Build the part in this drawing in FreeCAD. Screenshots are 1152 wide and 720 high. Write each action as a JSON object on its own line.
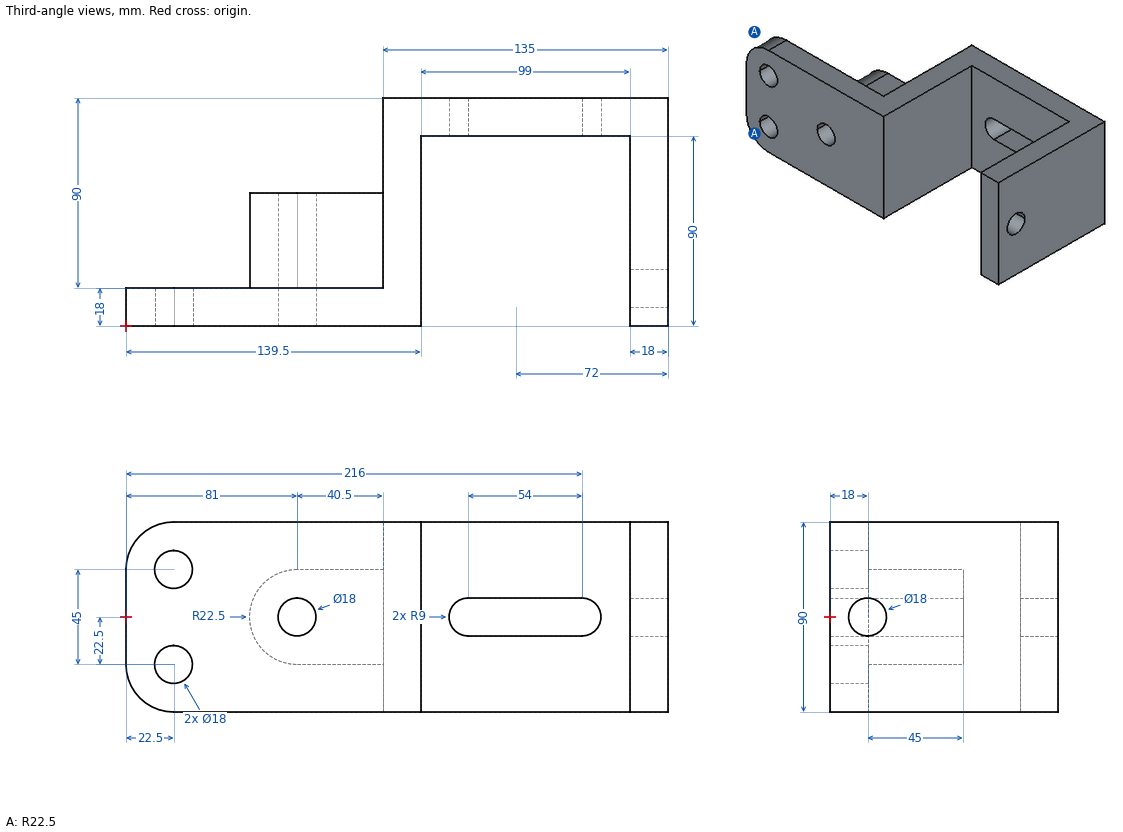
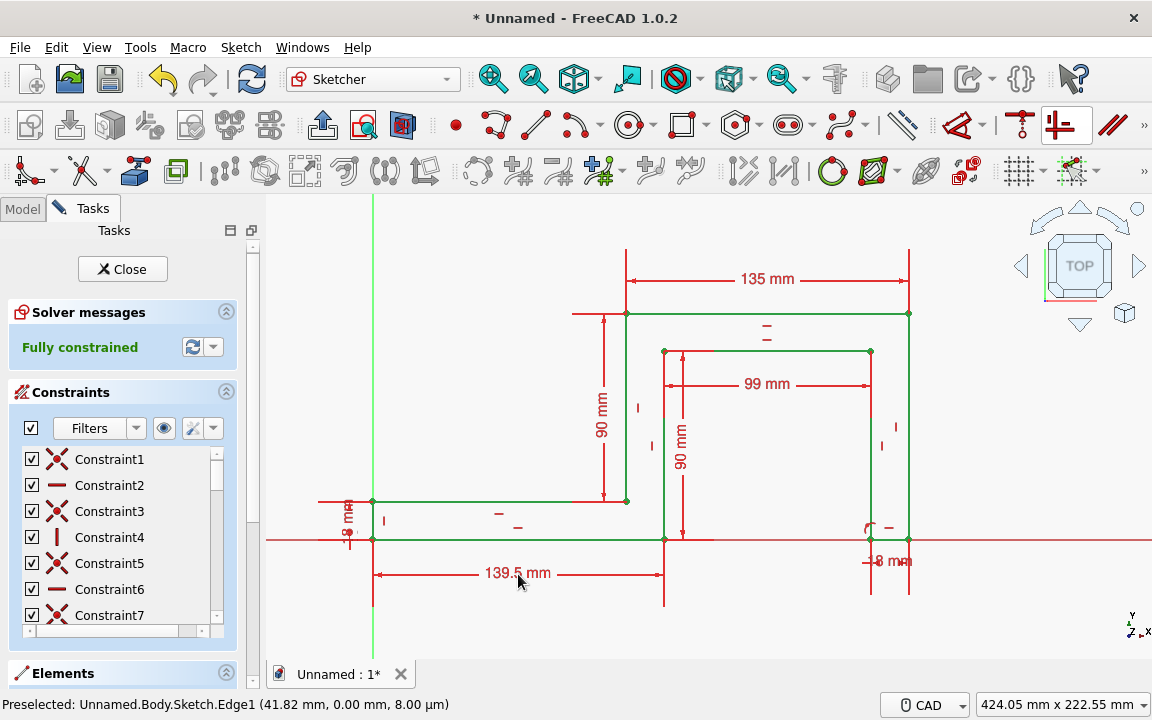
{"action": "left_click", "coordinate": [123, 269]}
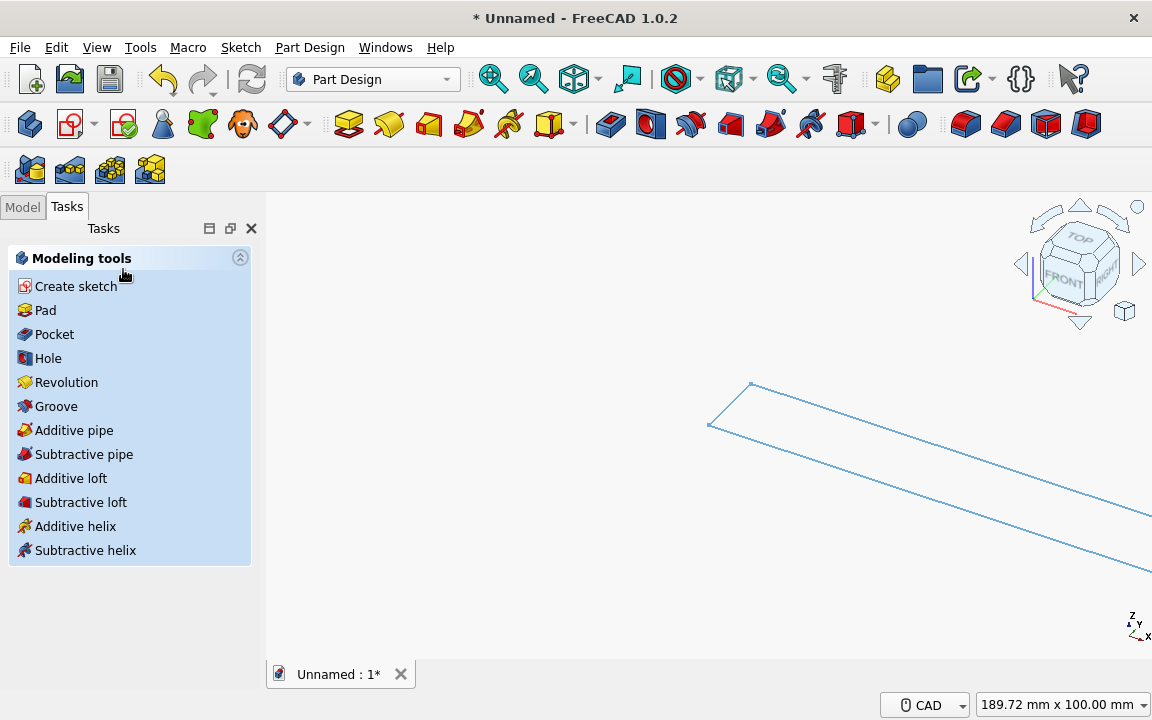
{"action": "left_click", "coordinate": [350, 124]}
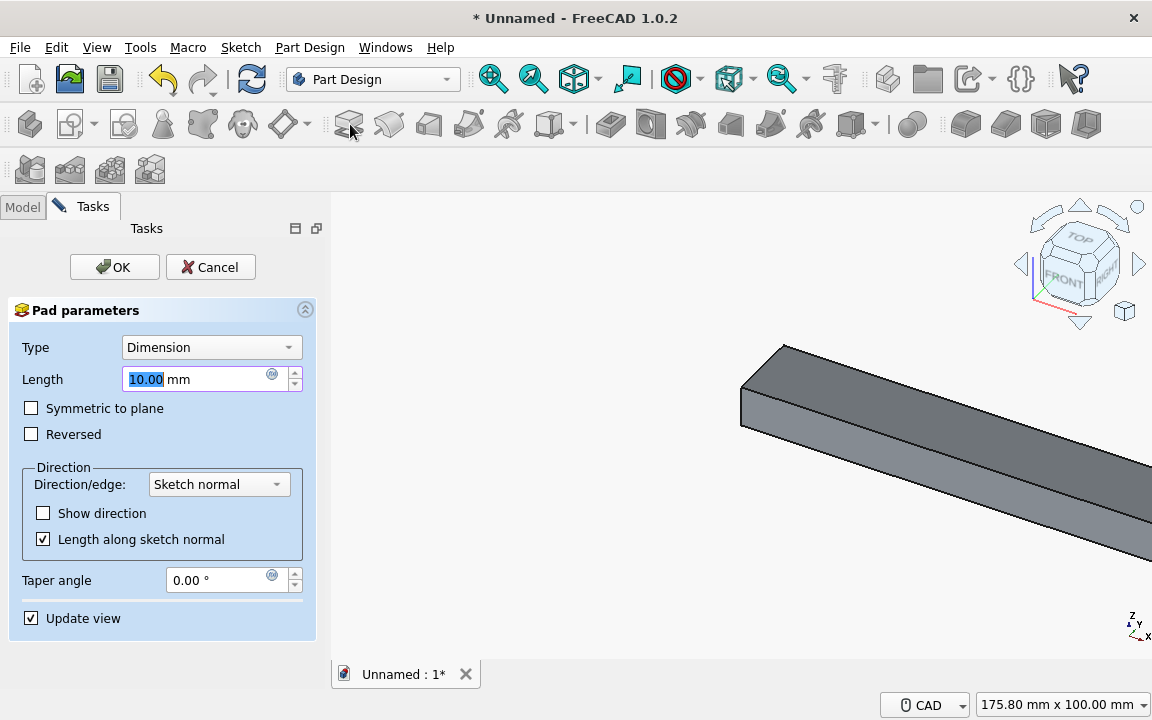
{"action": "type", "text": "90"}
{"action": "key", "text": "Tab"}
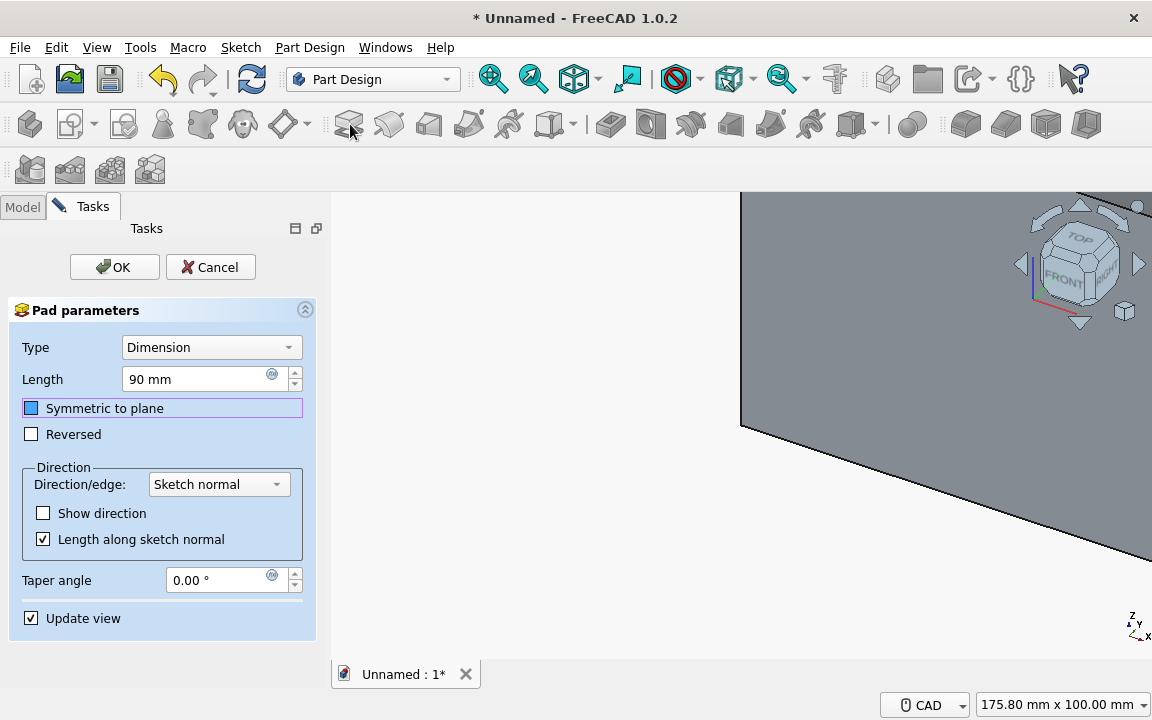
{"action": "left_click", "coordinate": [30, 408]}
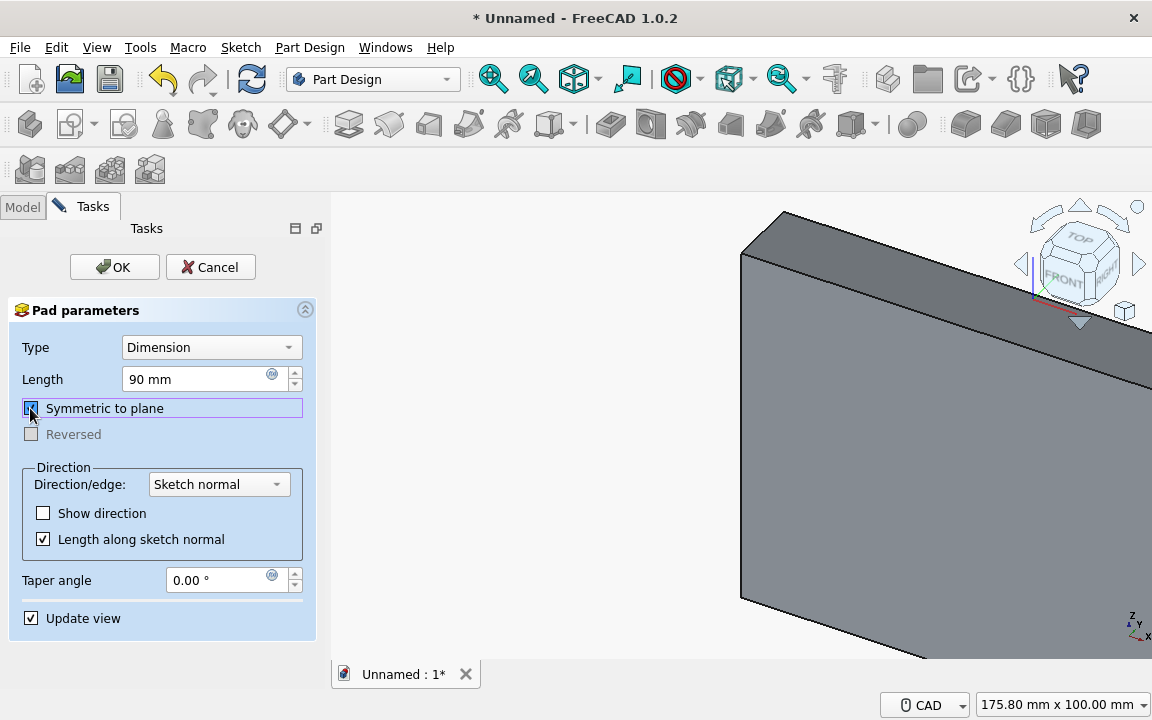
{"action": "left_click", "coordinate": [115, 267]}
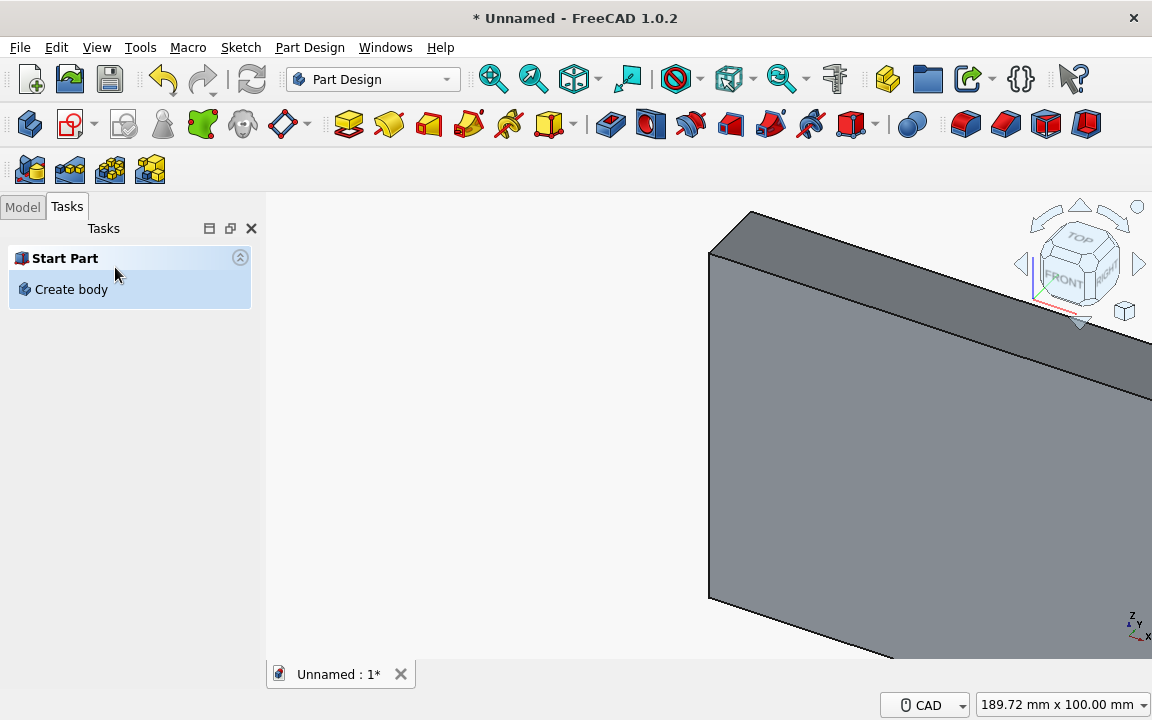
{"action": "left_click", "coordinate": [494, 80]}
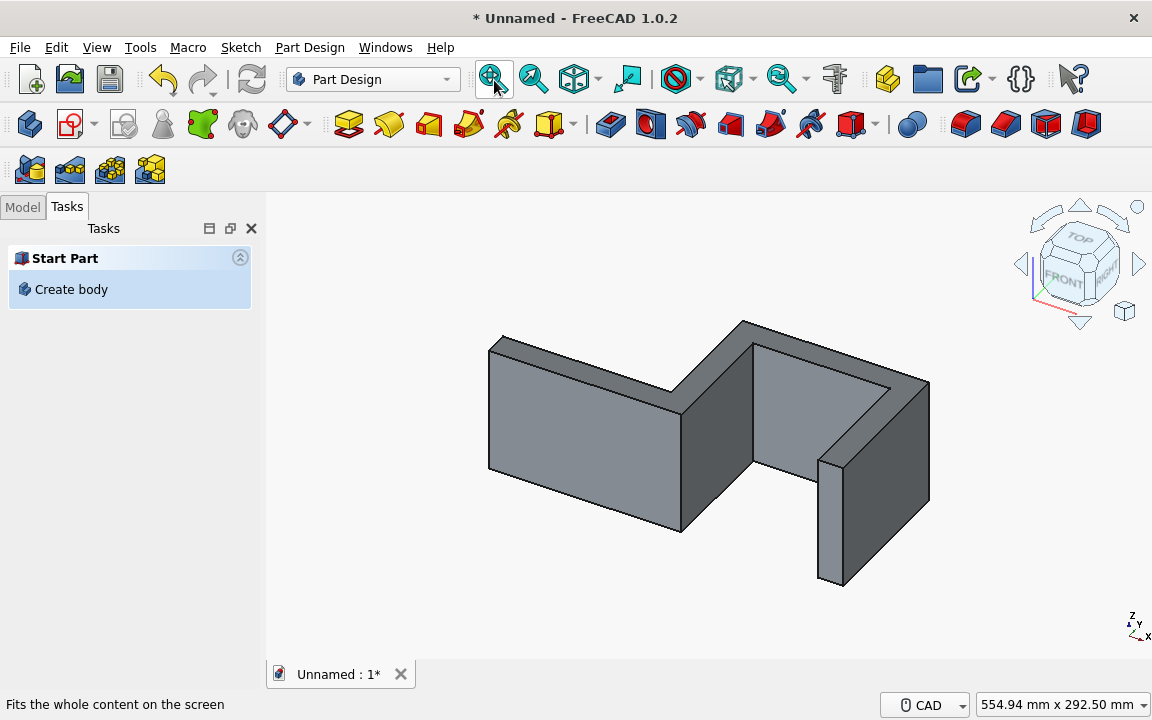
{"action": "key", "text": "4"}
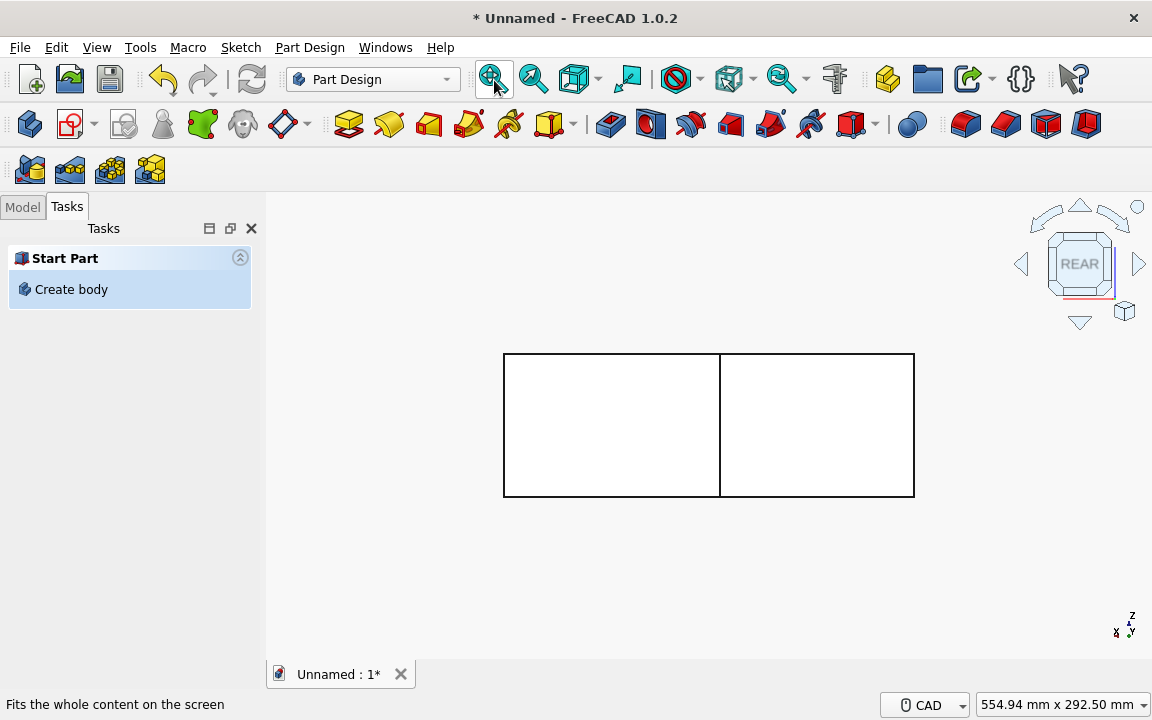
{"action": "left_click", "coordinate": [581, 424]}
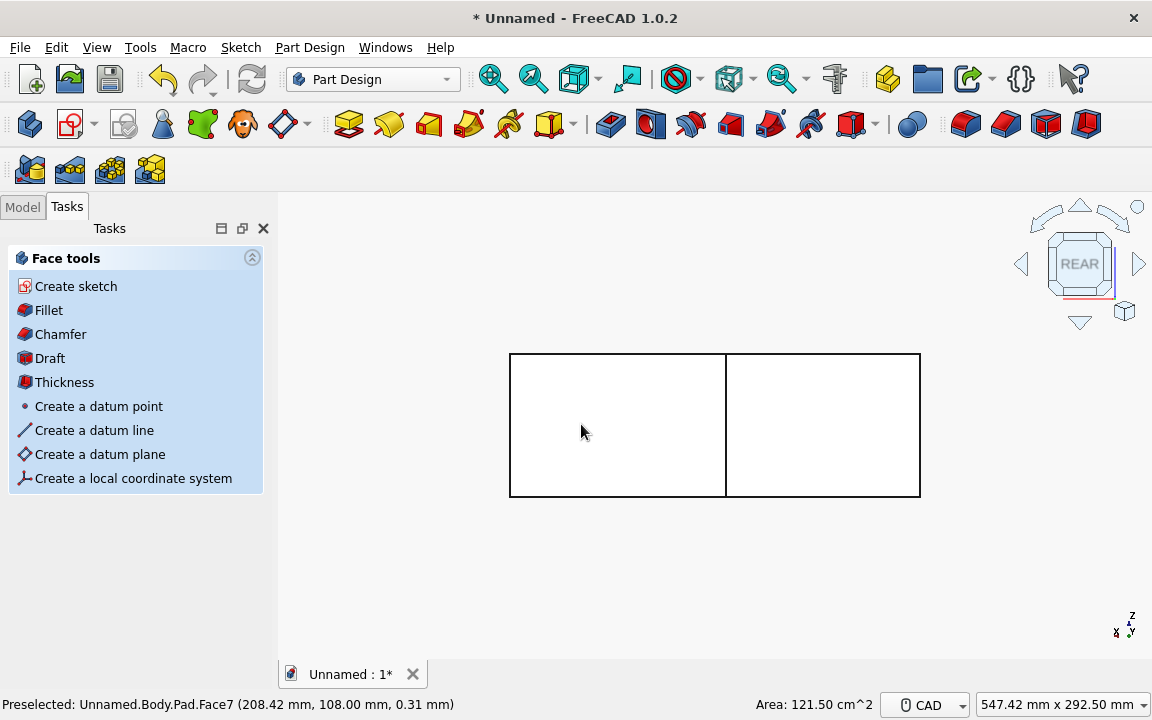
{"action": "left_click", "coordinate": [70, 124]}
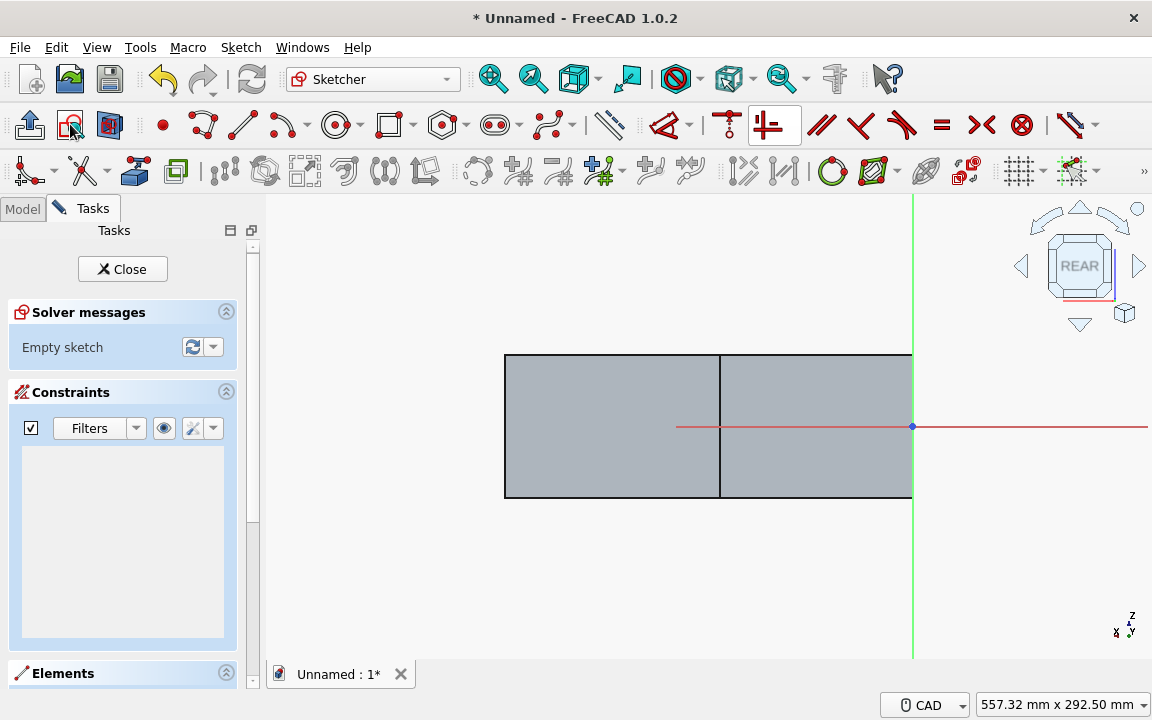
{"action": "scroll", "coordinate": [603, 426], "scroll_direction": "up", "scroll_amount": 7}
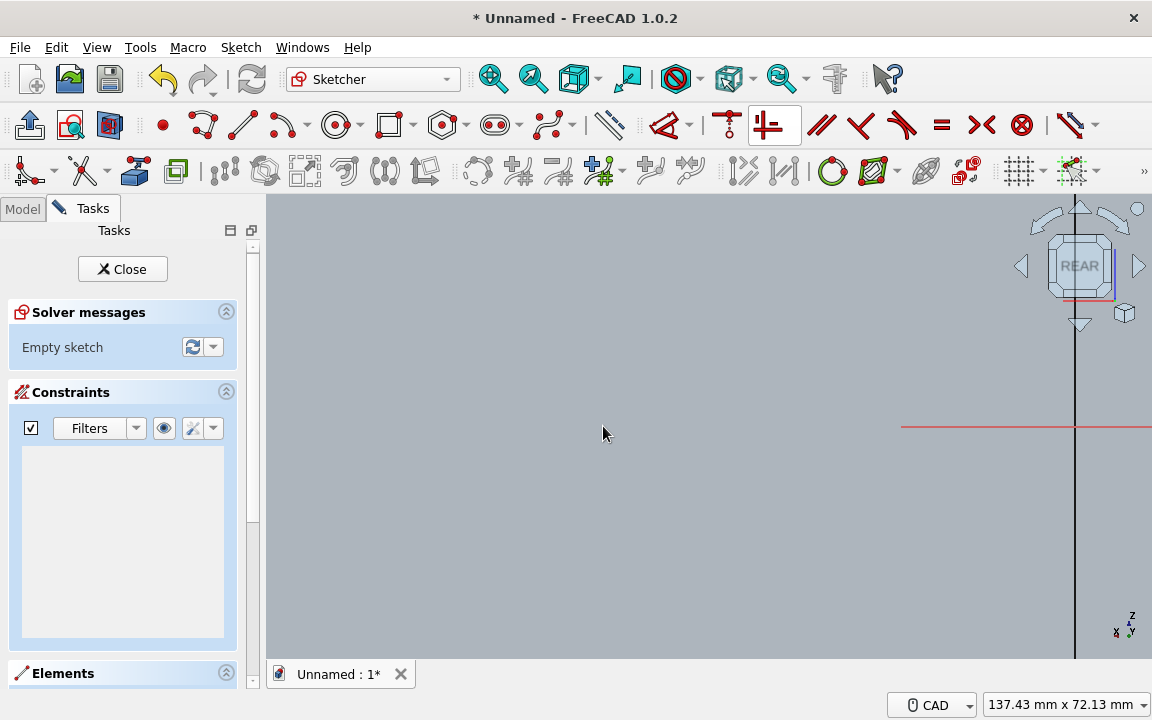
{"action": "left_click", "coordinate": [496, 126]}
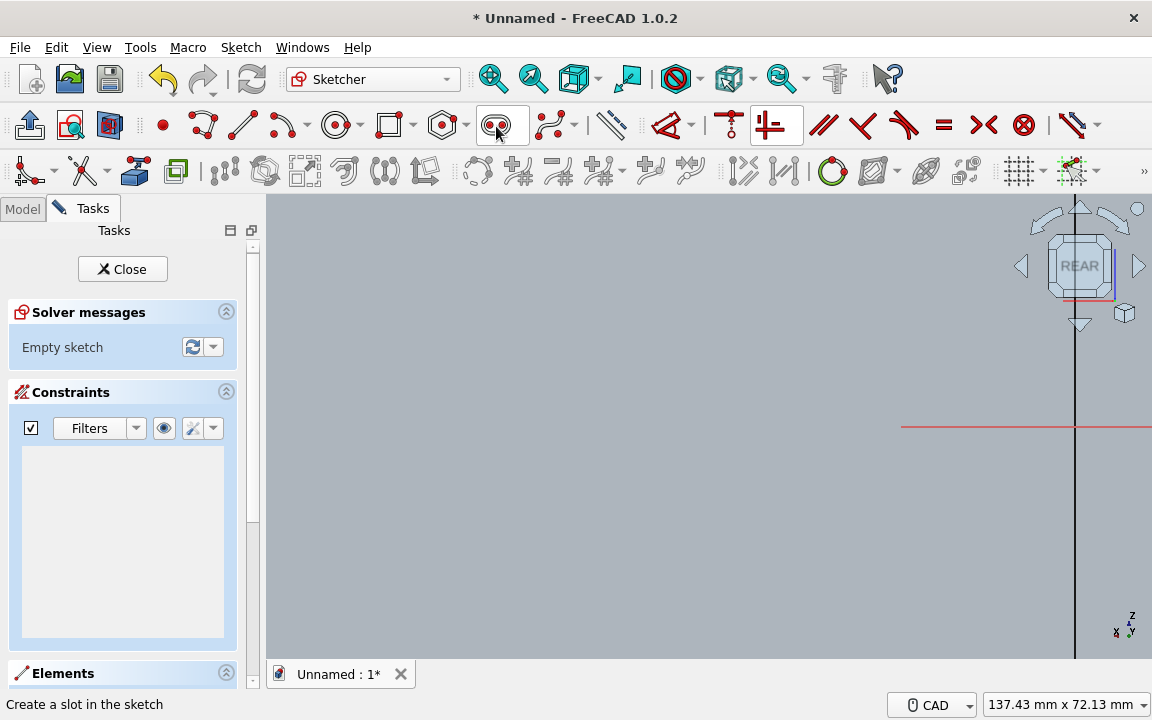
{"action": "left_click", "coordinate": [466, 426]}